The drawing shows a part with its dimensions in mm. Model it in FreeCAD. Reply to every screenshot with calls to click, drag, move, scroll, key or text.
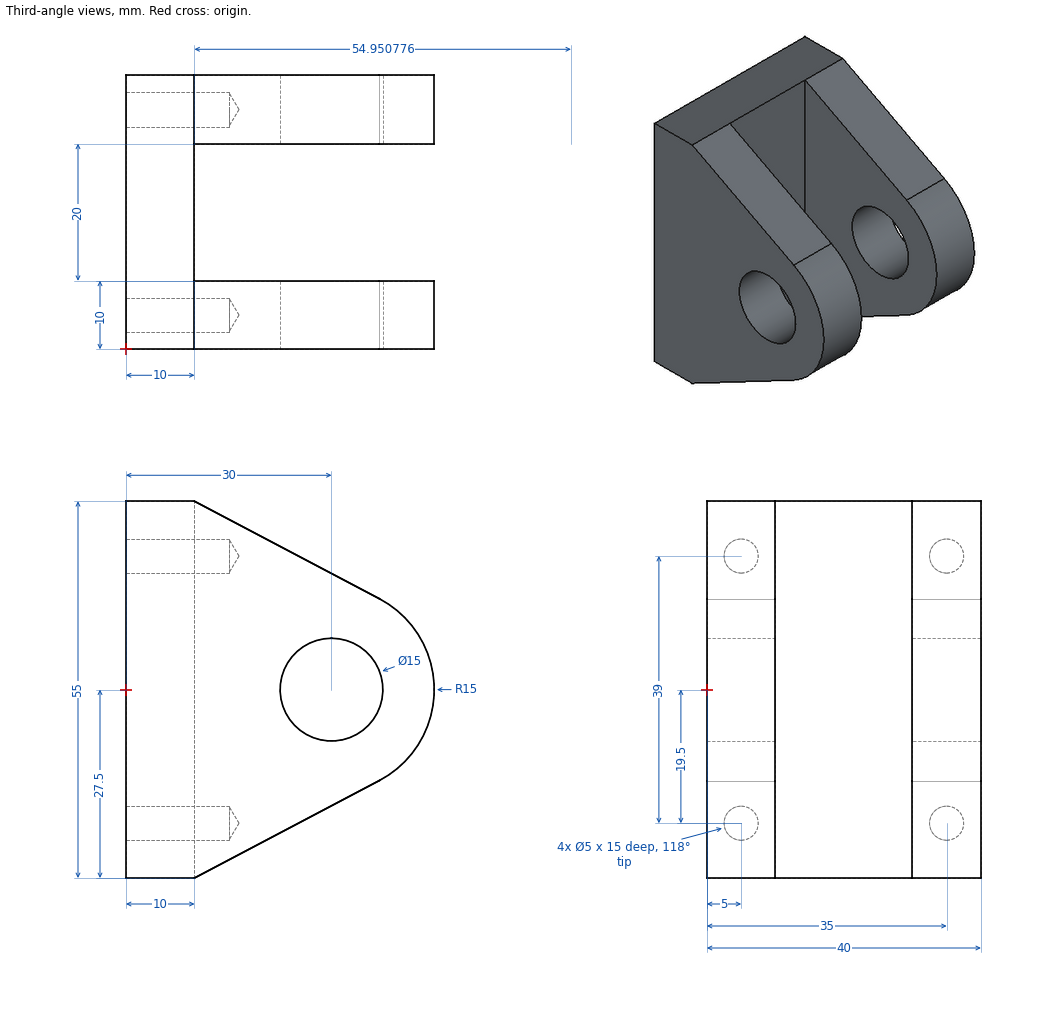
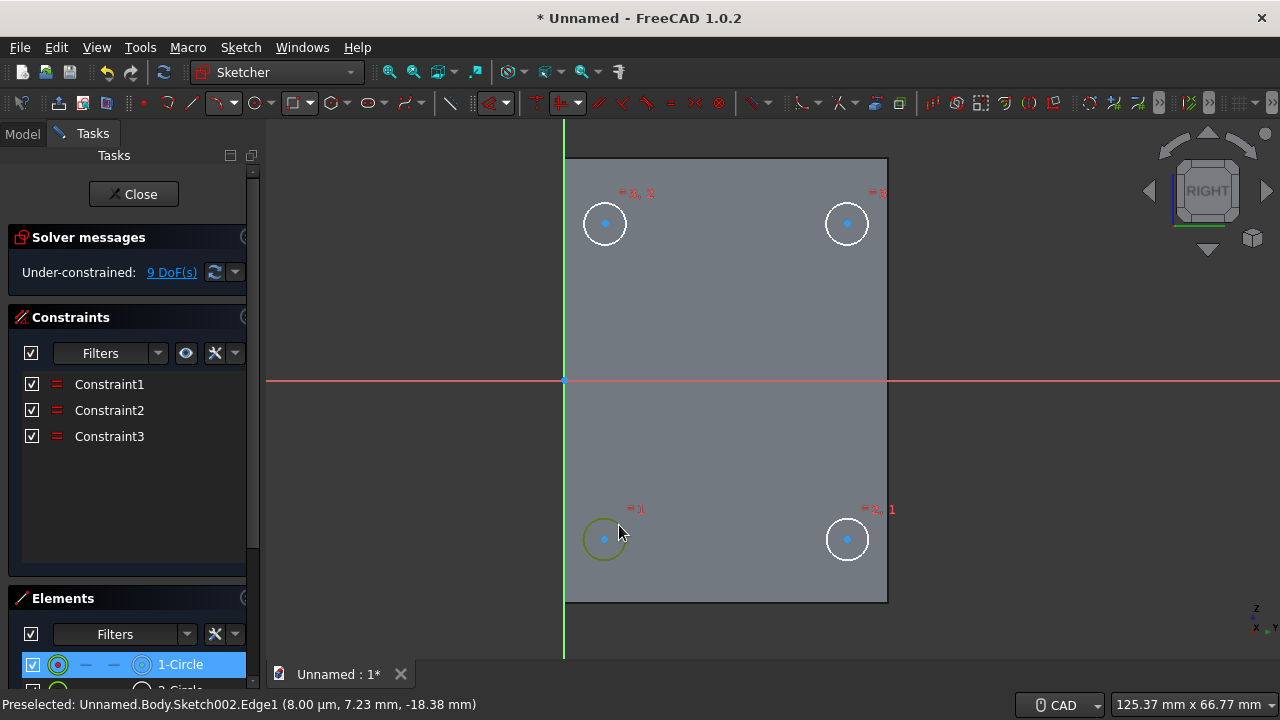
key(k)
key(o)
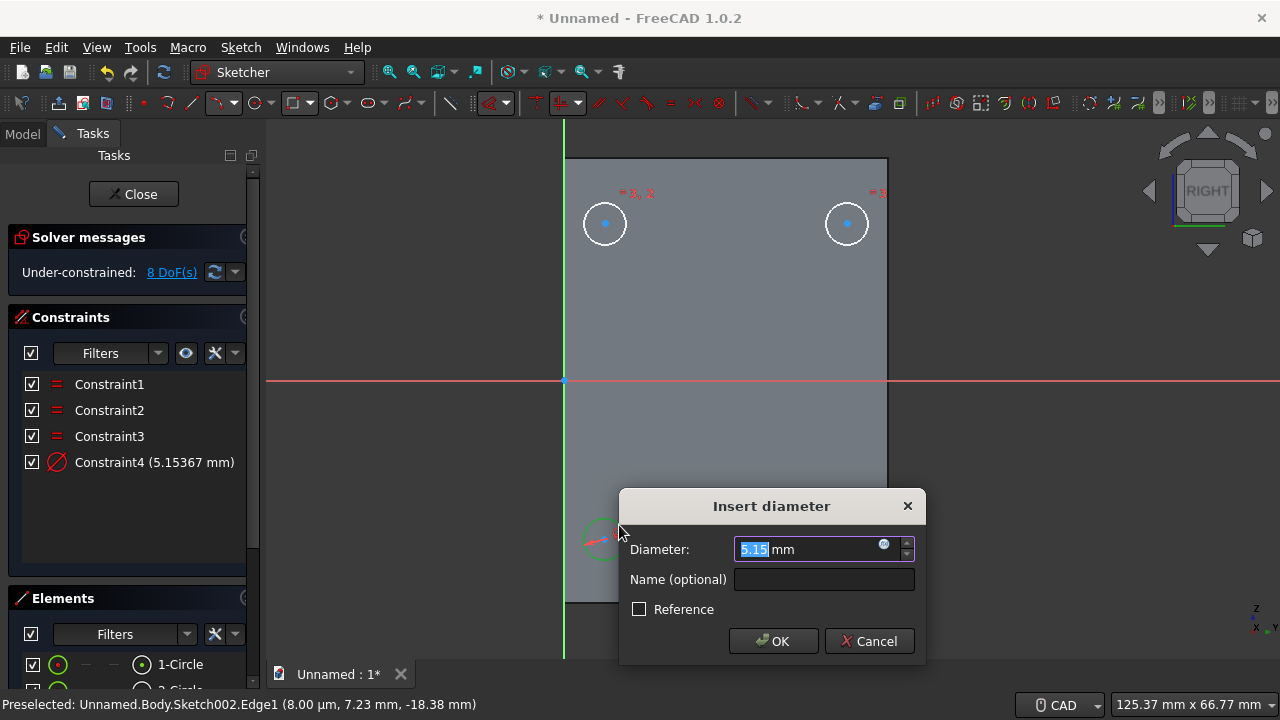
text(5)
key(Return)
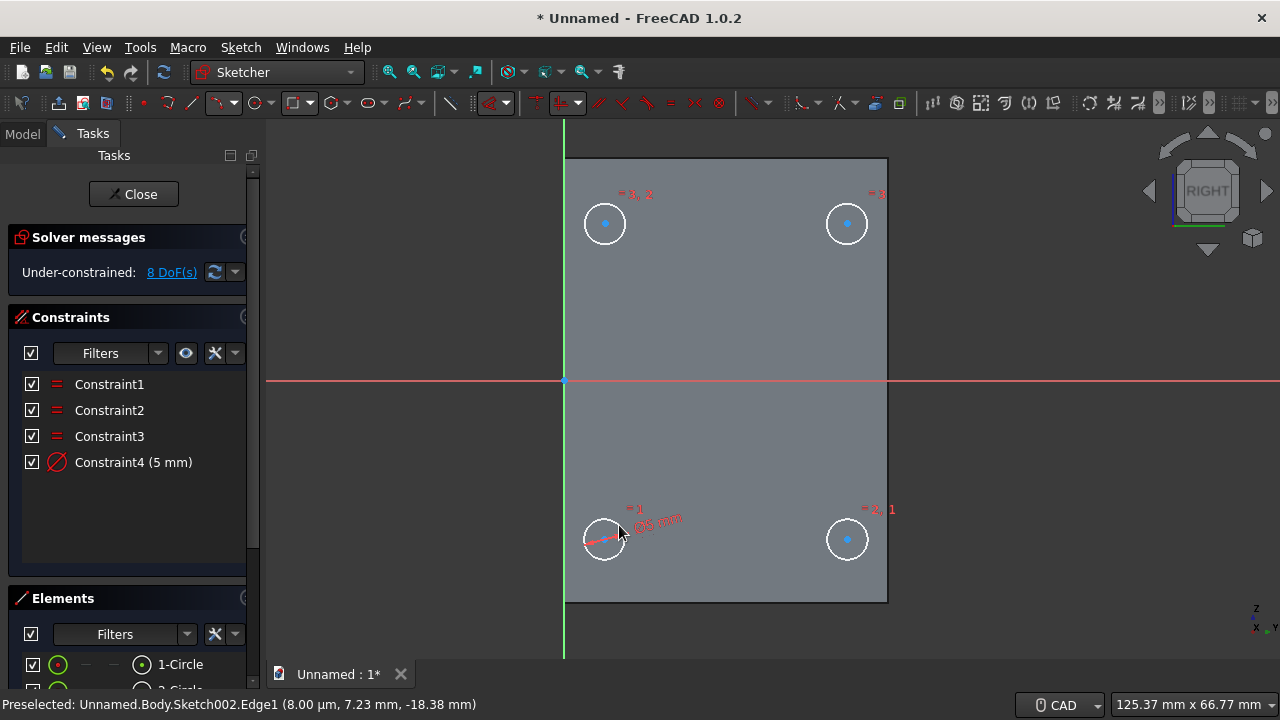
click(604, 539)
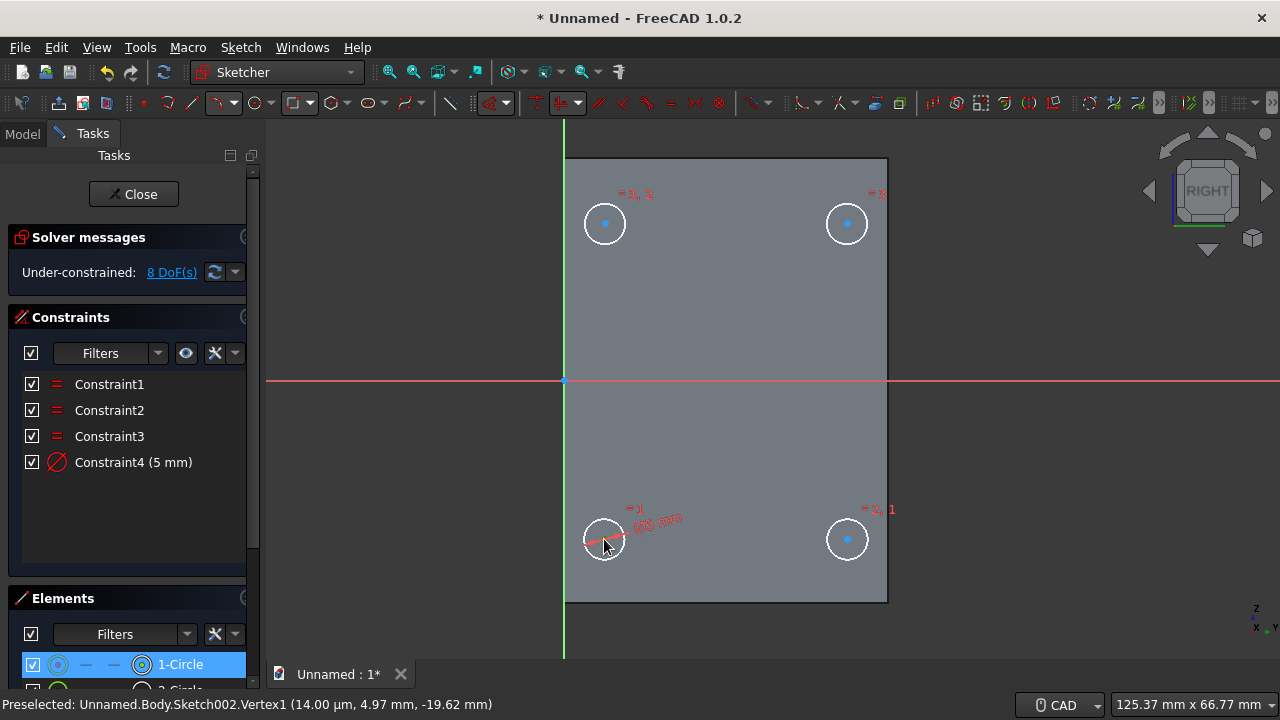
key(l)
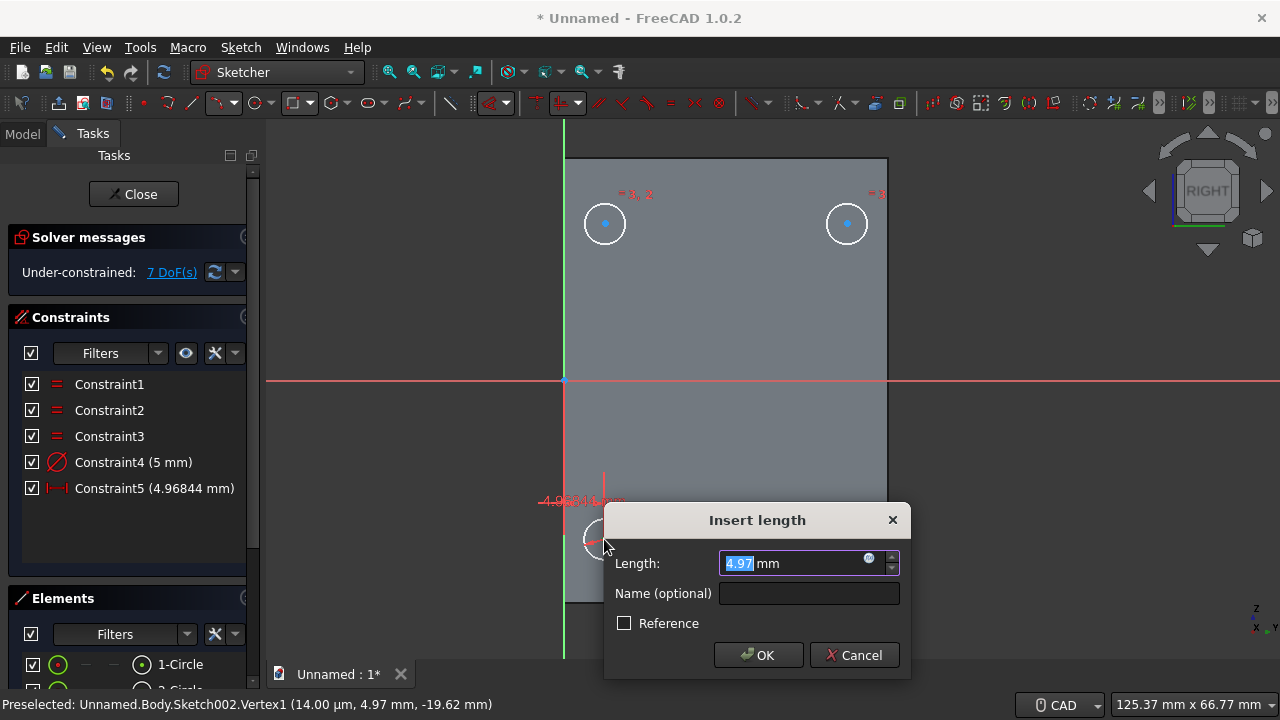
text(5)
key(Return)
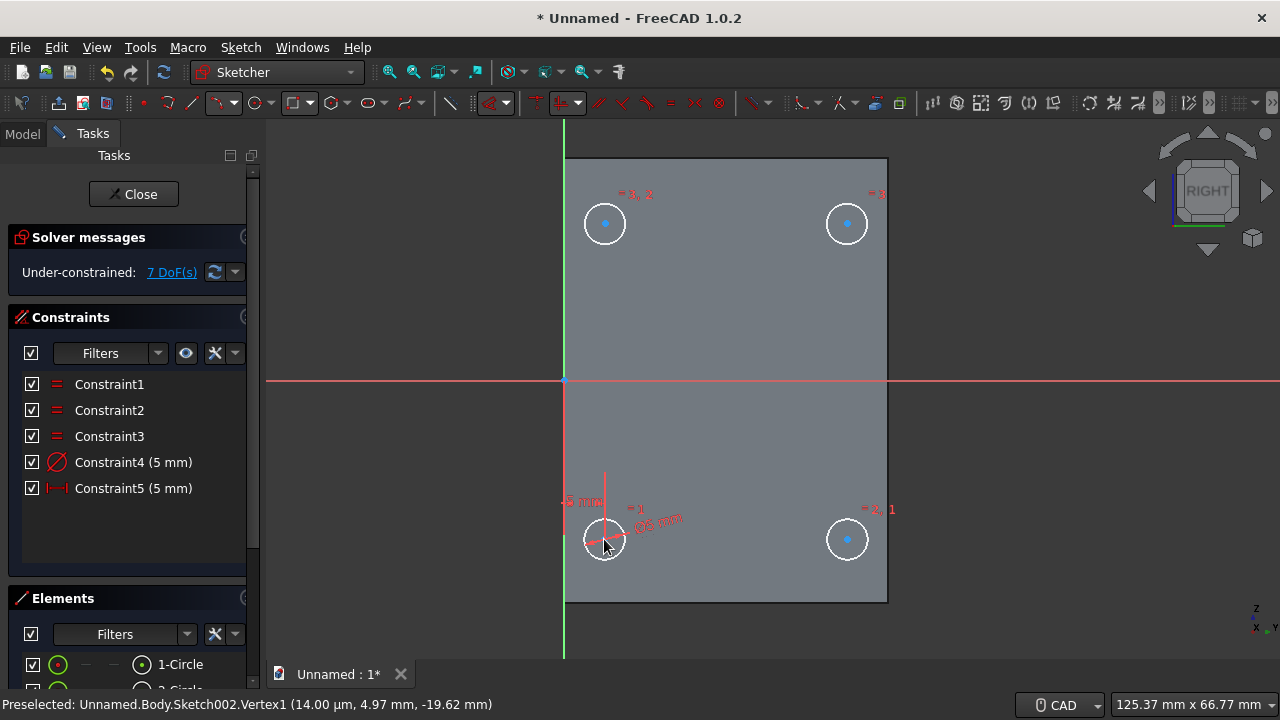
click(605, 224)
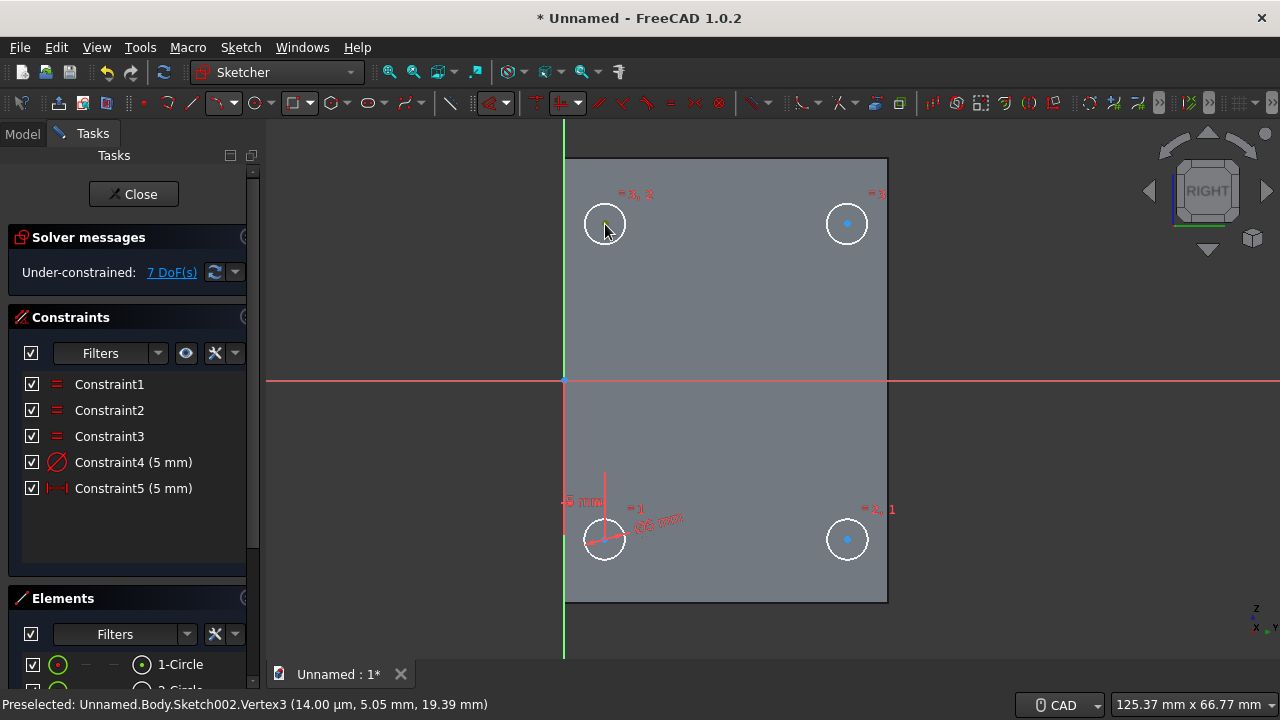
key(l)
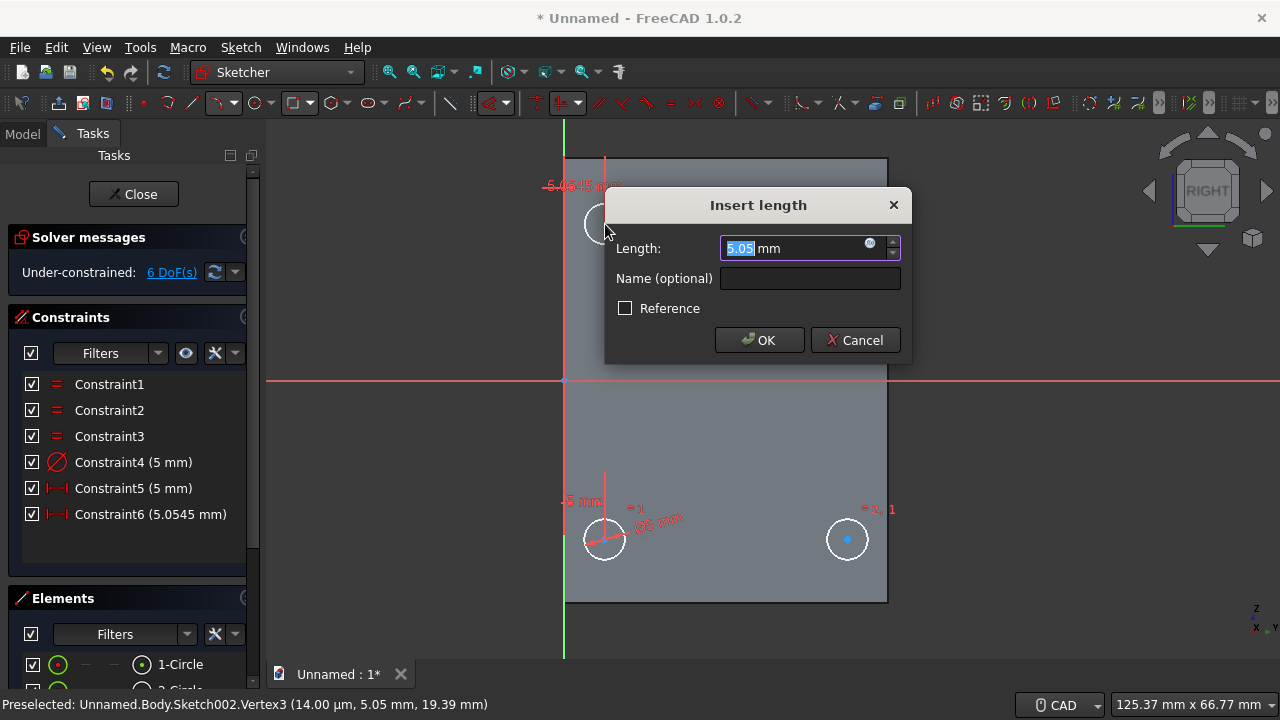
text(5)
key(Return)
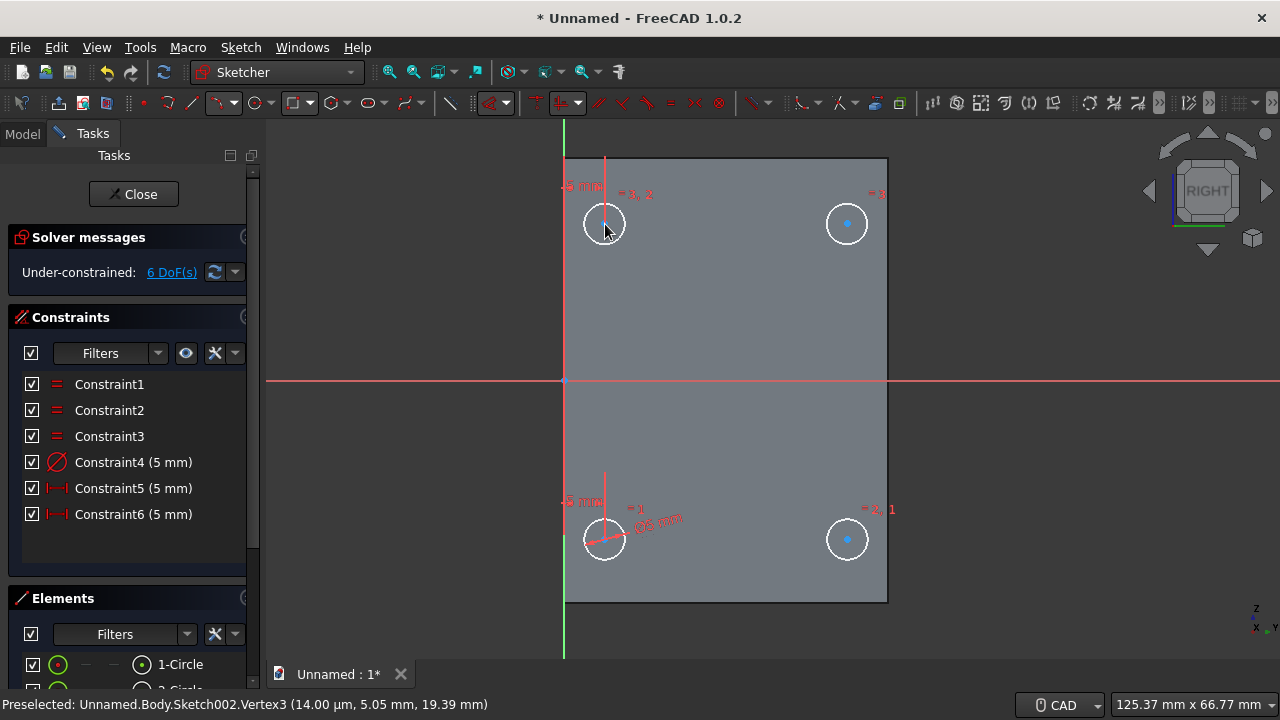
click(847, 539)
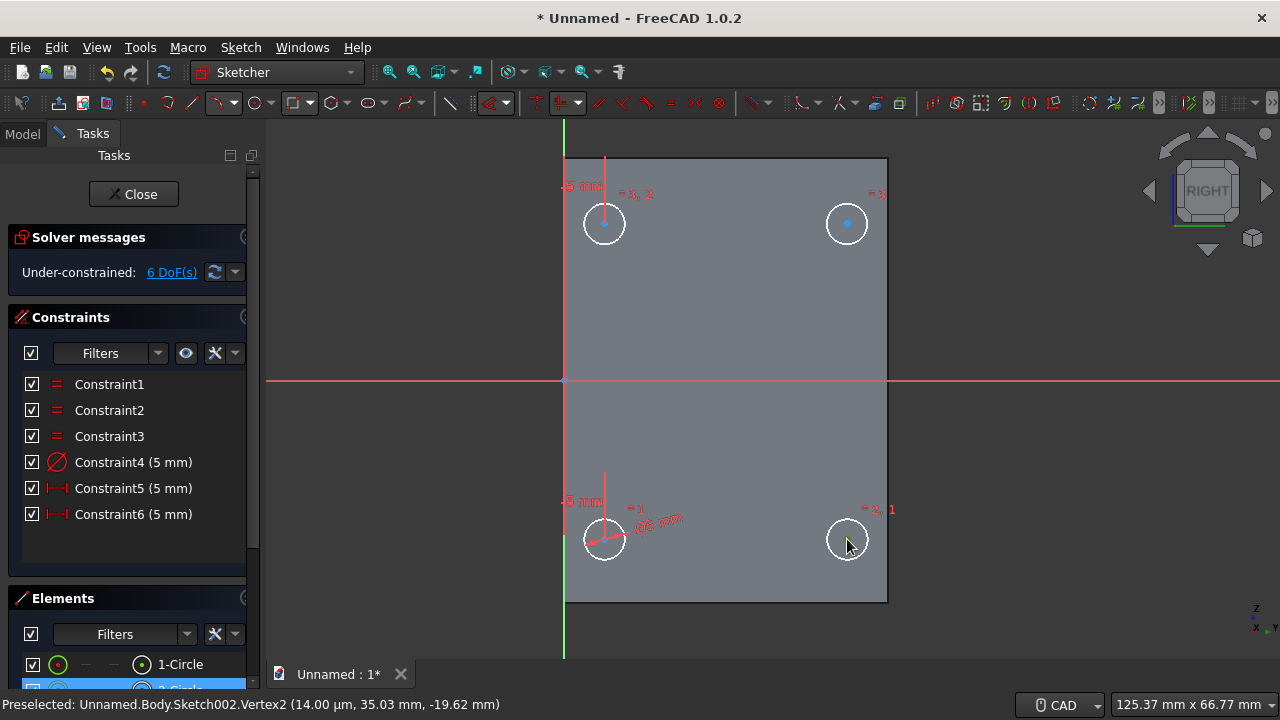
key(l)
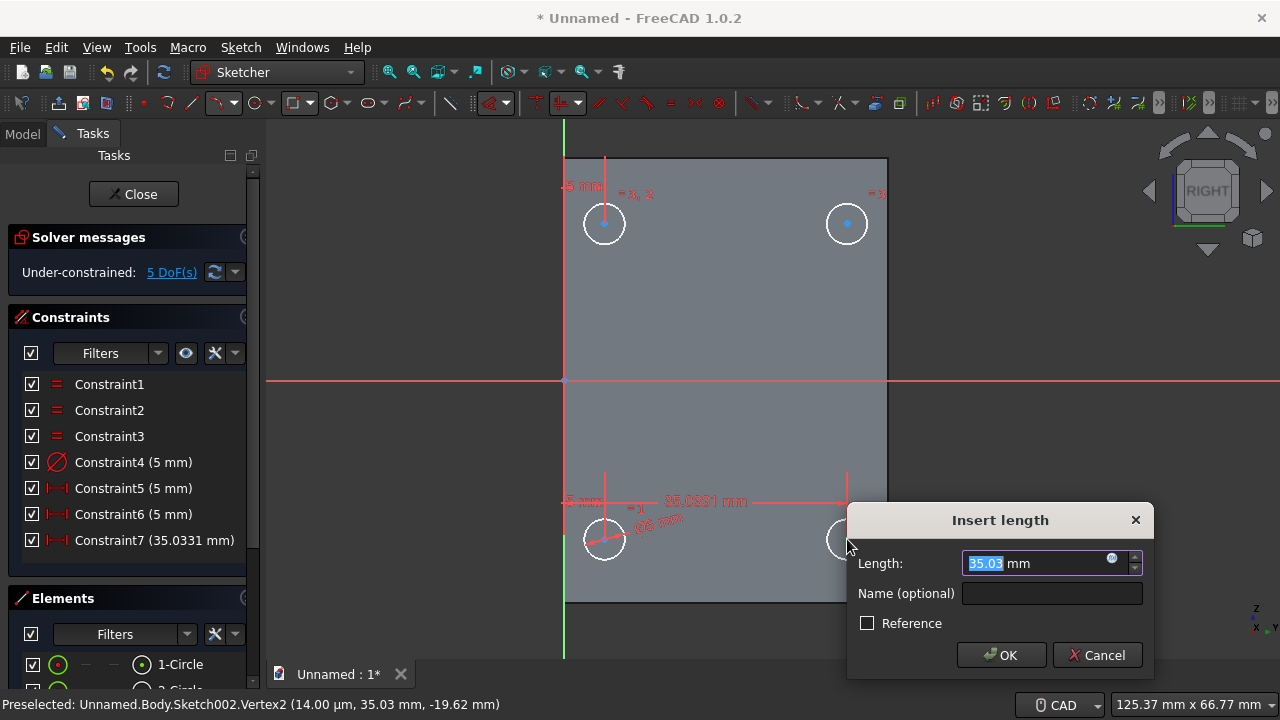
text(35)
key(Return)